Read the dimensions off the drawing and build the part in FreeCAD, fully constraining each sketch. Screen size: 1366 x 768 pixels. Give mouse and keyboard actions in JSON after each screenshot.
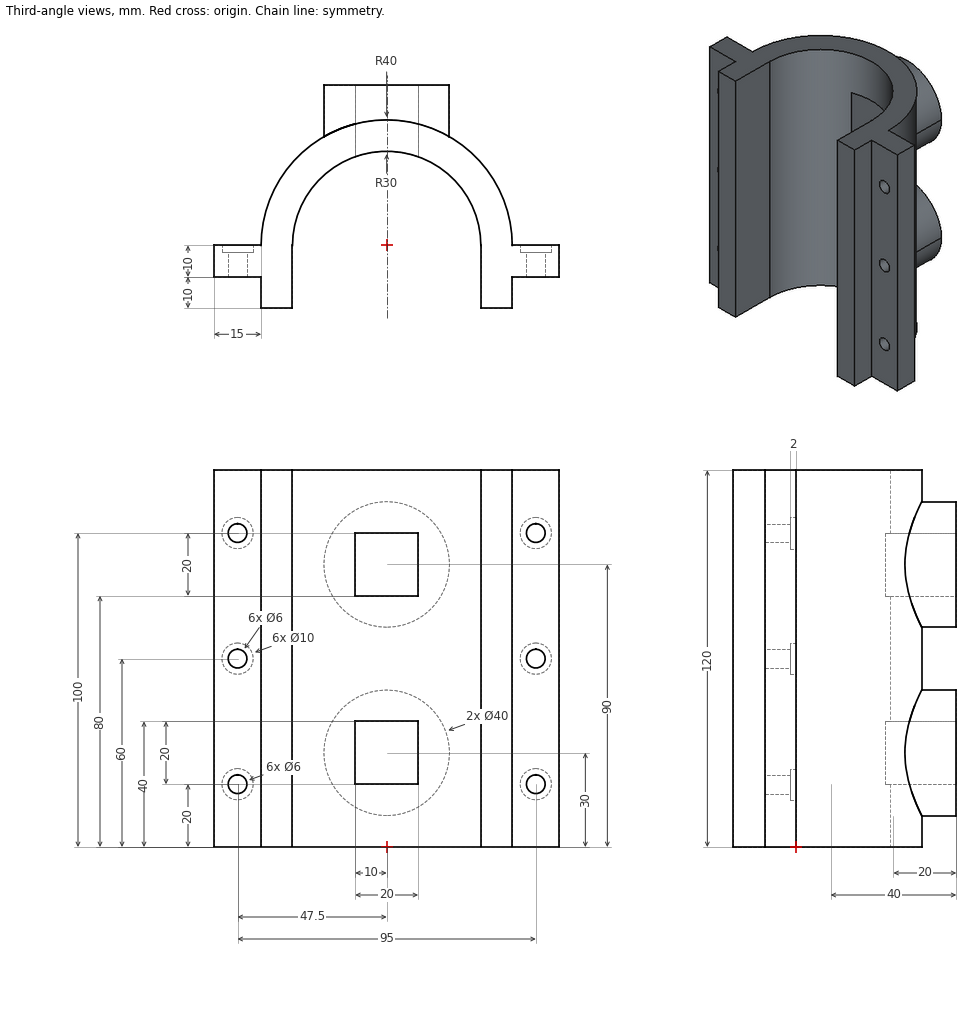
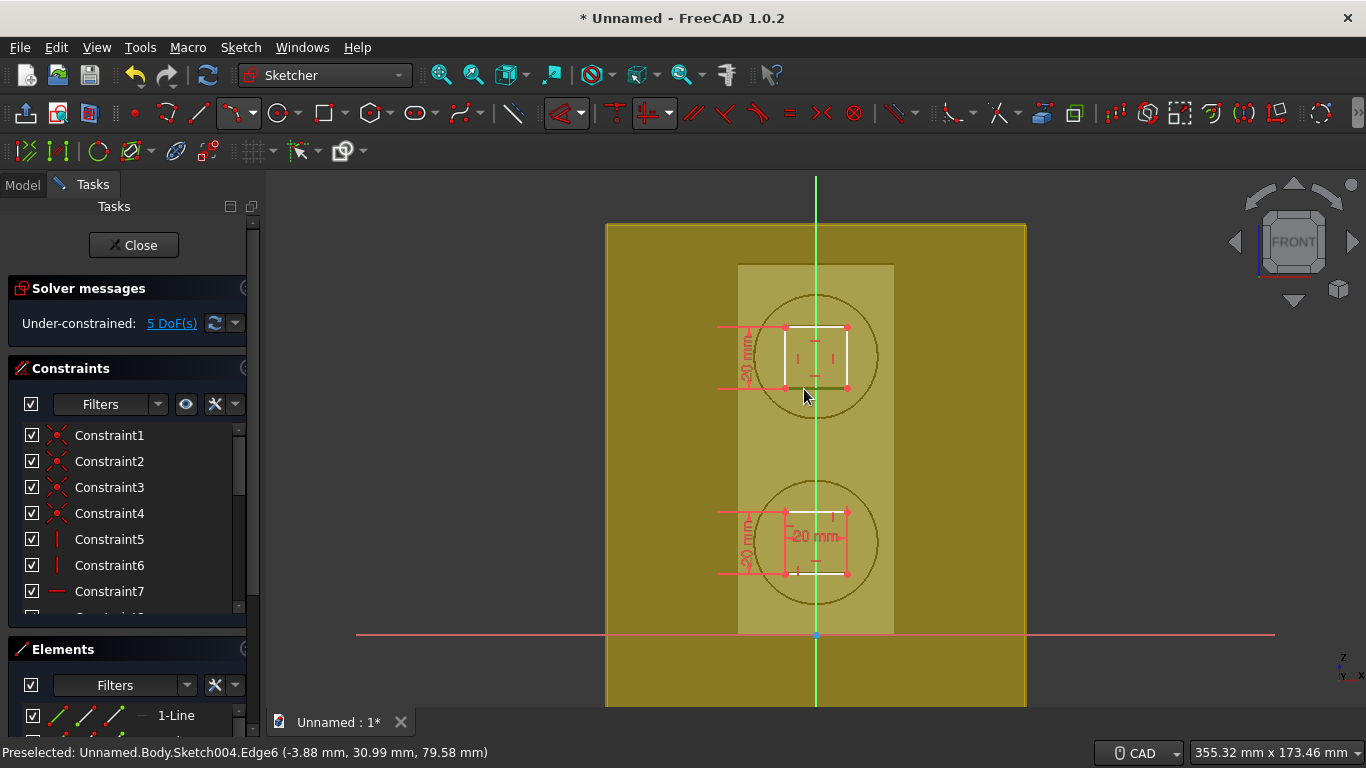
{"action": "key", "text": "l"}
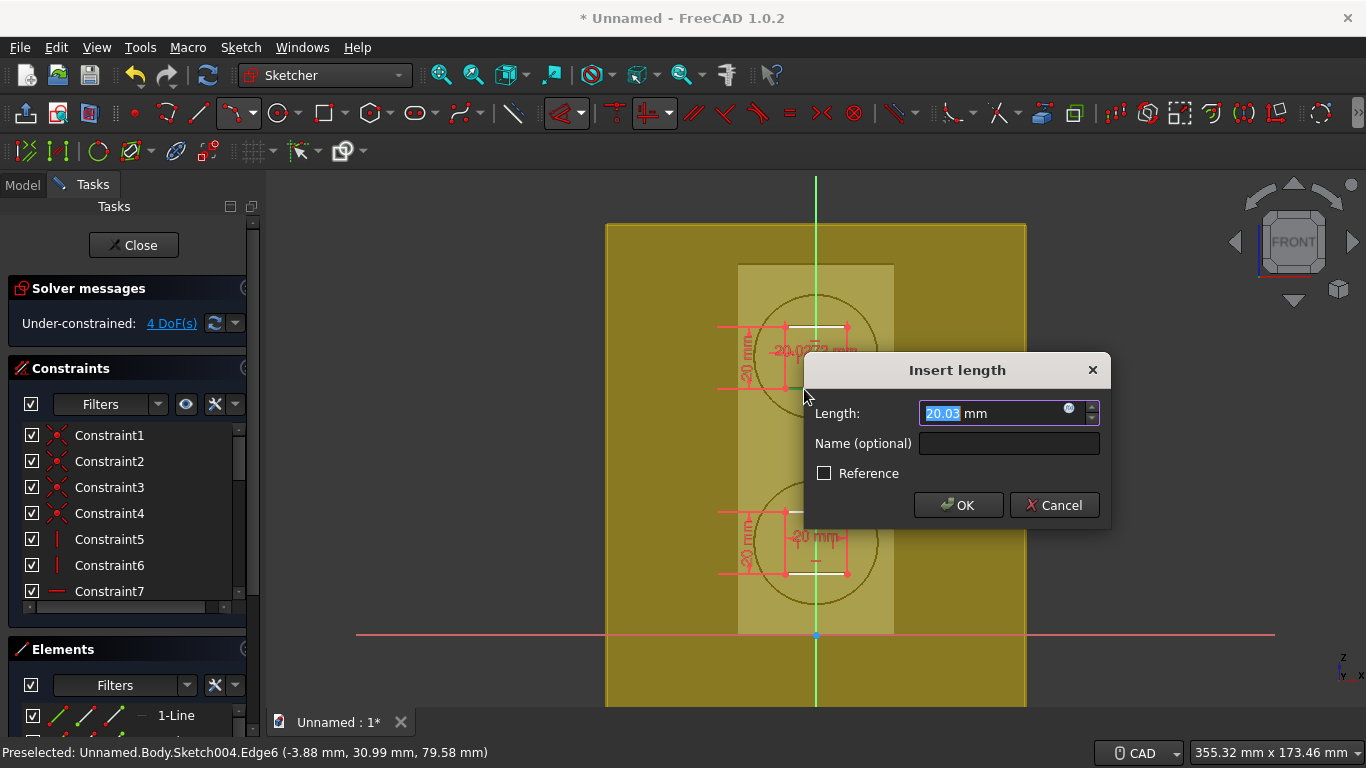
{"action": "type", "text": "20"}
{"action": "key", "text": "Return"}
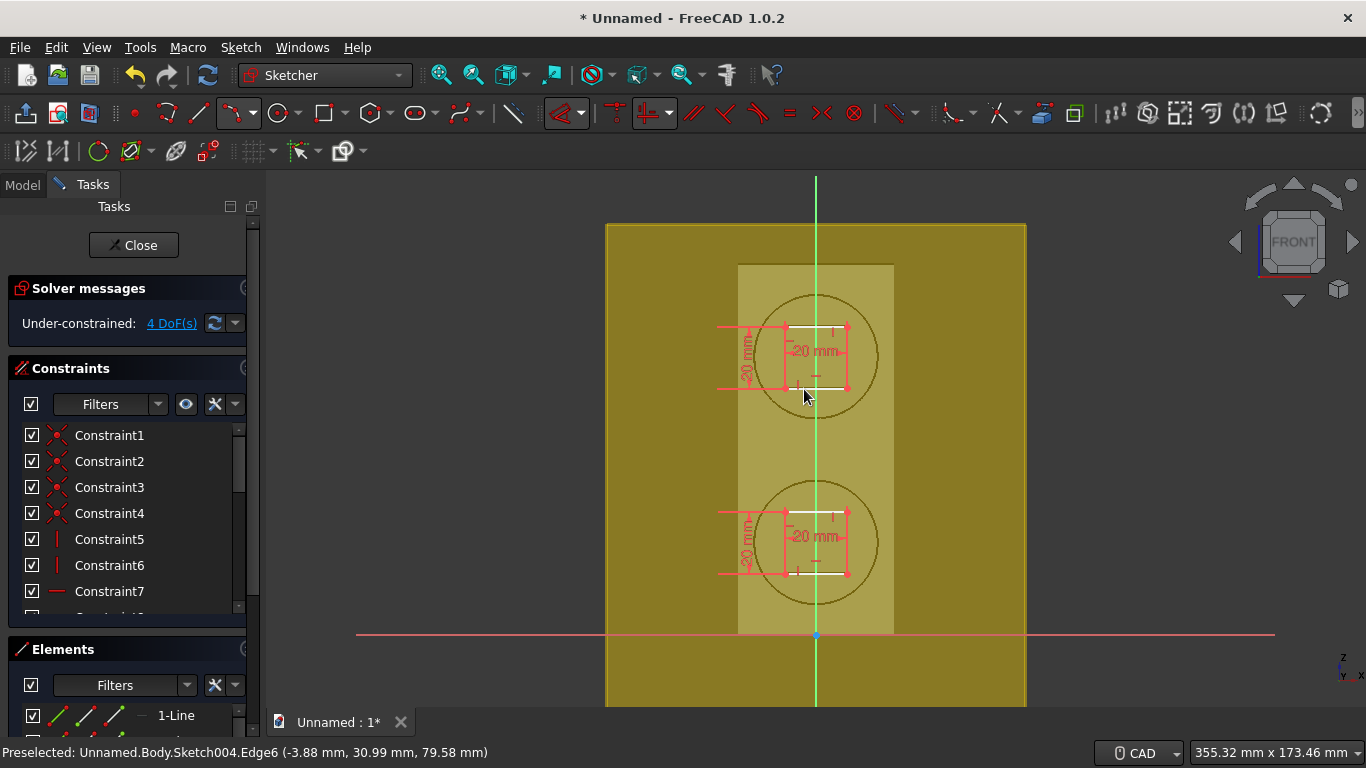
{"action": "scroll", "coordinate": [785, 512], "scroll_direction": "up", "scroll_amount": 2}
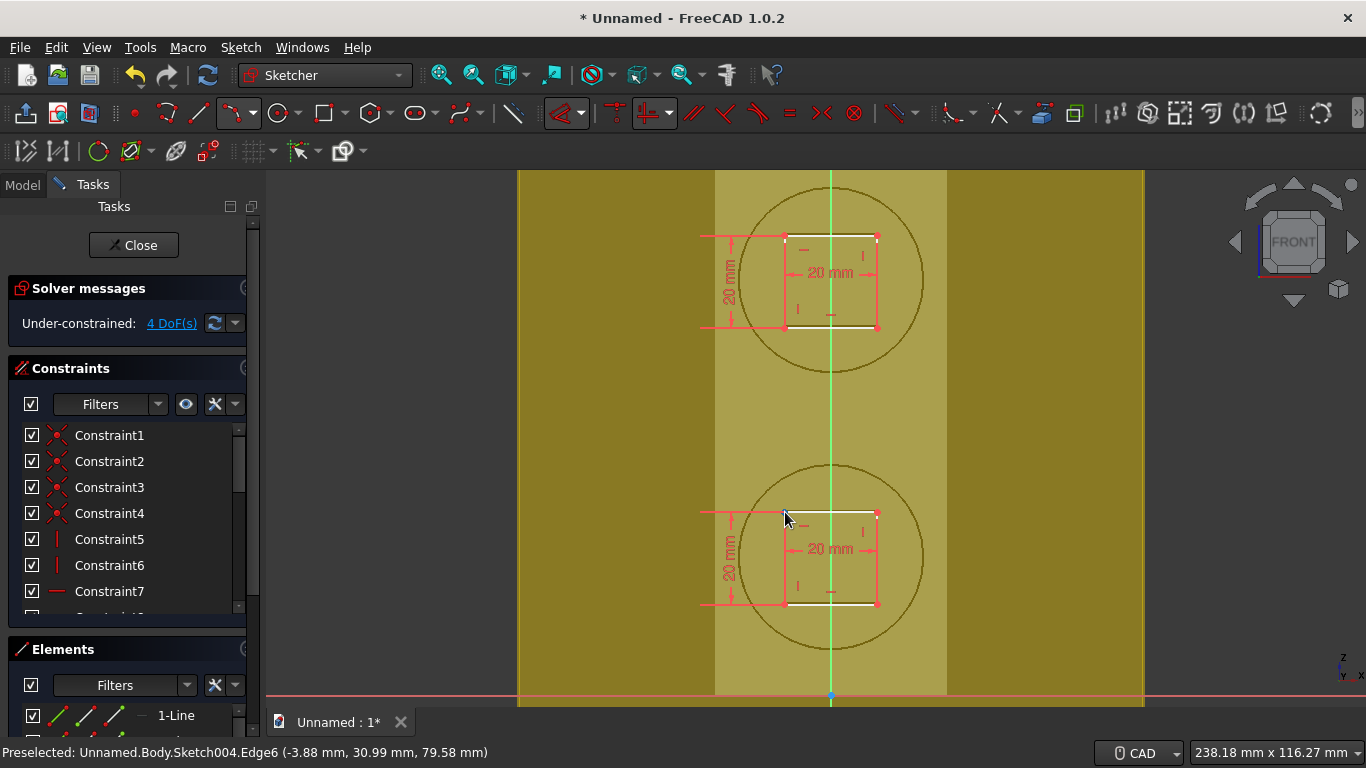
{"action": "left_click", "coordinate": [785, 512]}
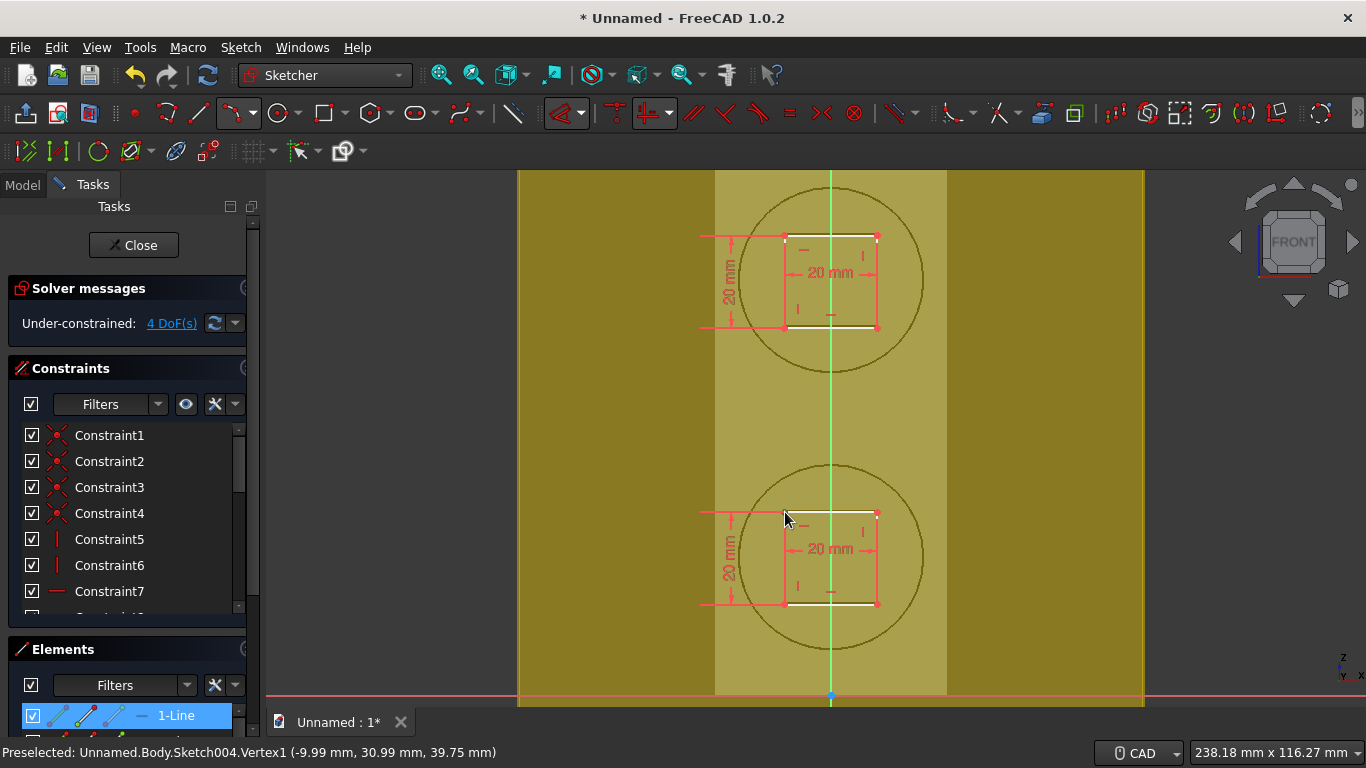
{"action": "key", "text": "l"}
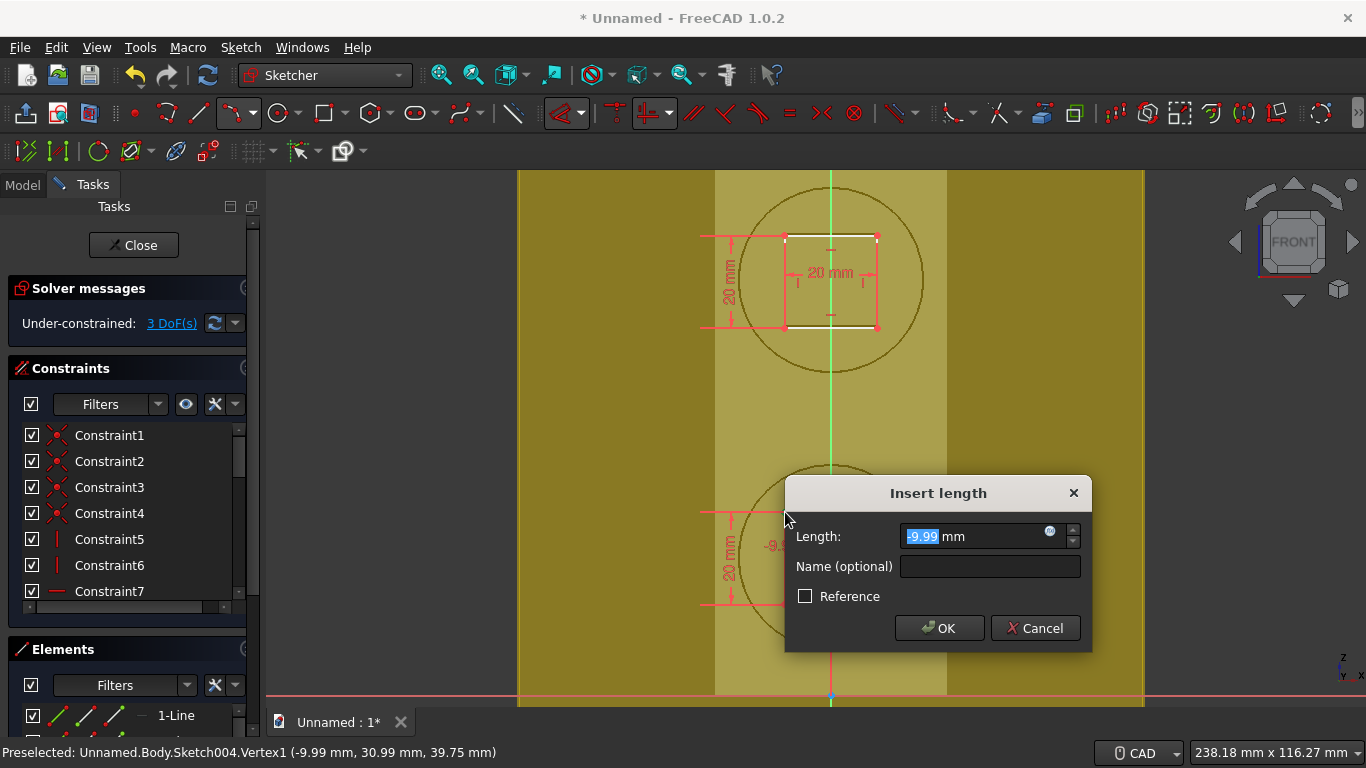
{"action": "type", "text": "-10"}
{"action": "key", "text": "Return"}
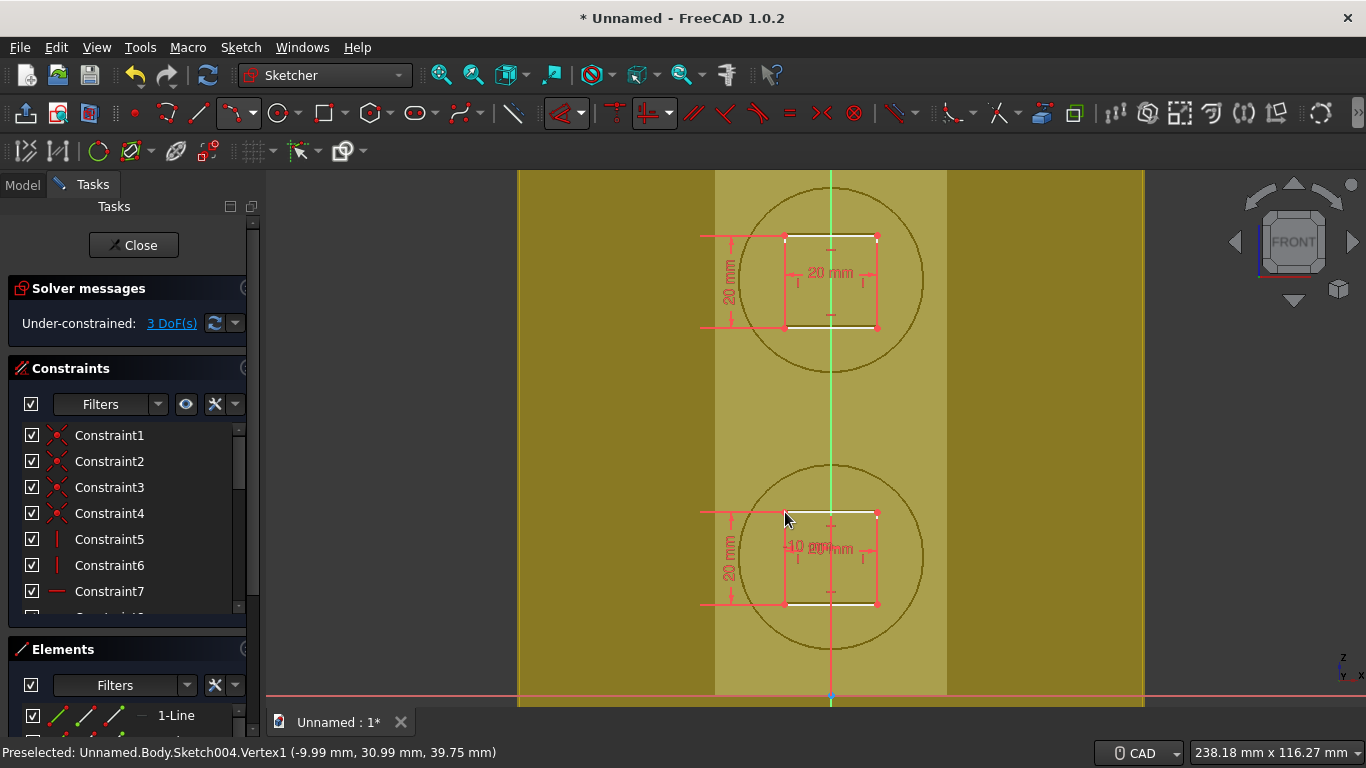
{"action": "left_click", "coordinate": [785, 512]}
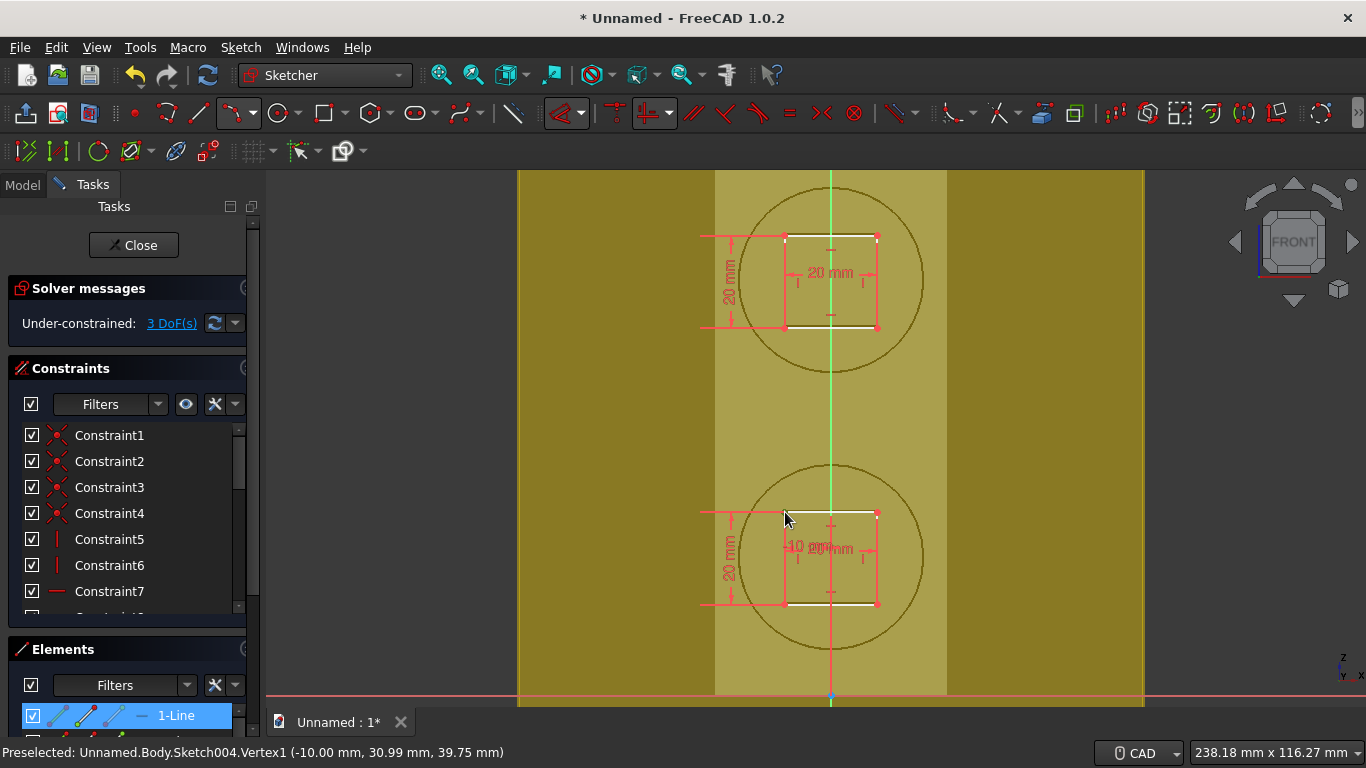
{"action": "left_click", "coordinate": [584, 114]}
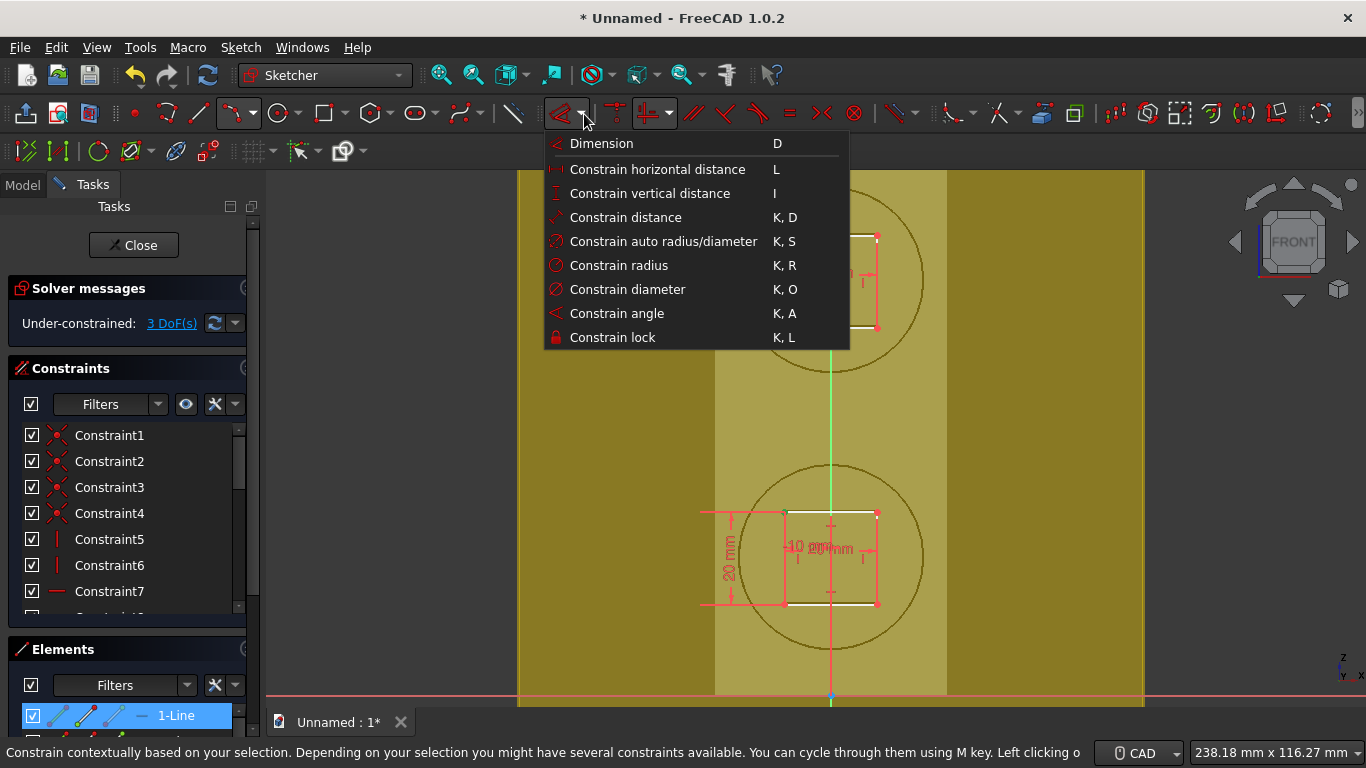
{"action": "left_click", "coordinate": [697, 193]}